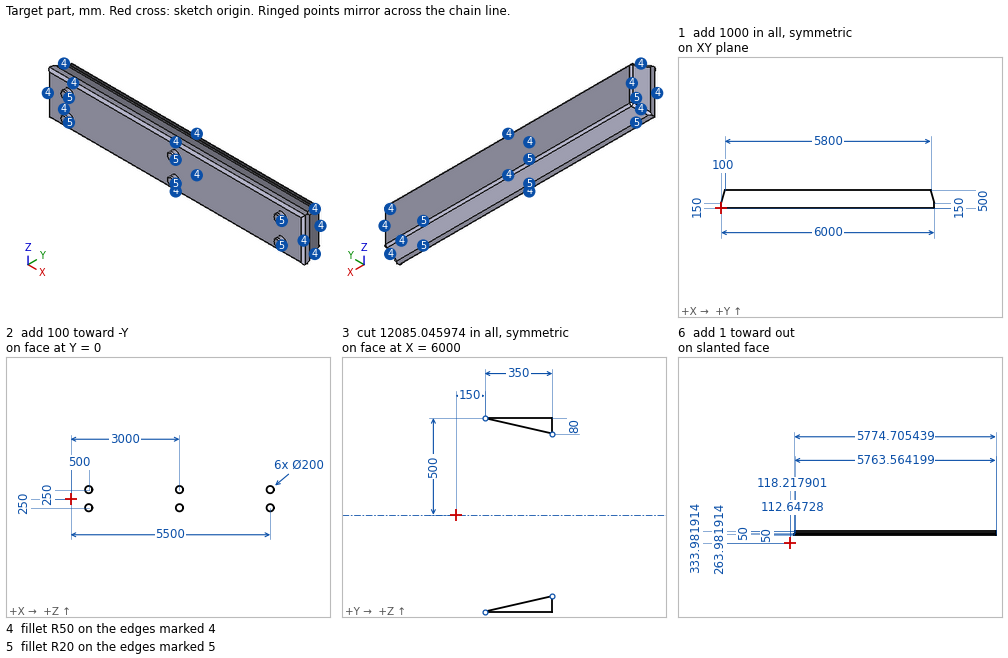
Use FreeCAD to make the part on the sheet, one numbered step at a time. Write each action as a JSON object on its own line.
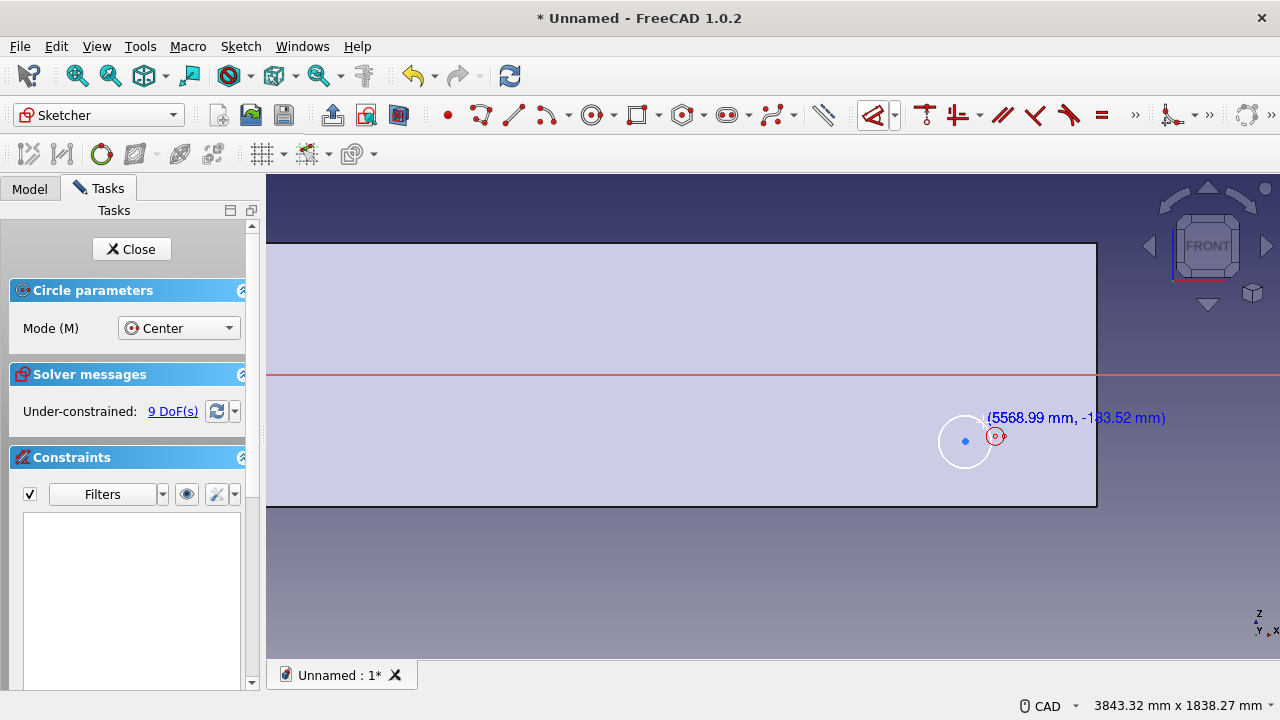
{"action": "left_click", "coordinate": [965, 309]}
{"action": "left_click", "coordinate": [983, 290]}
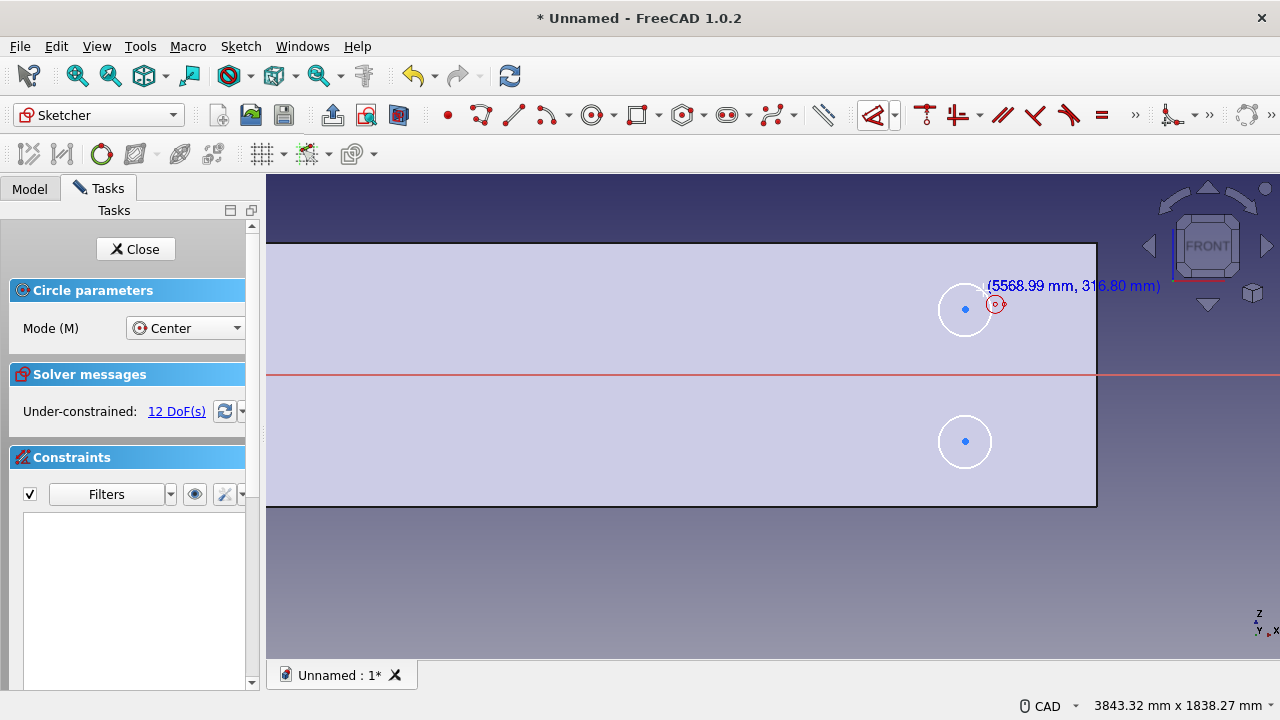
{"action": "left_click", "coordinate": [305, 309]}
{"action": "left_click", "coordinate": [324, 290]}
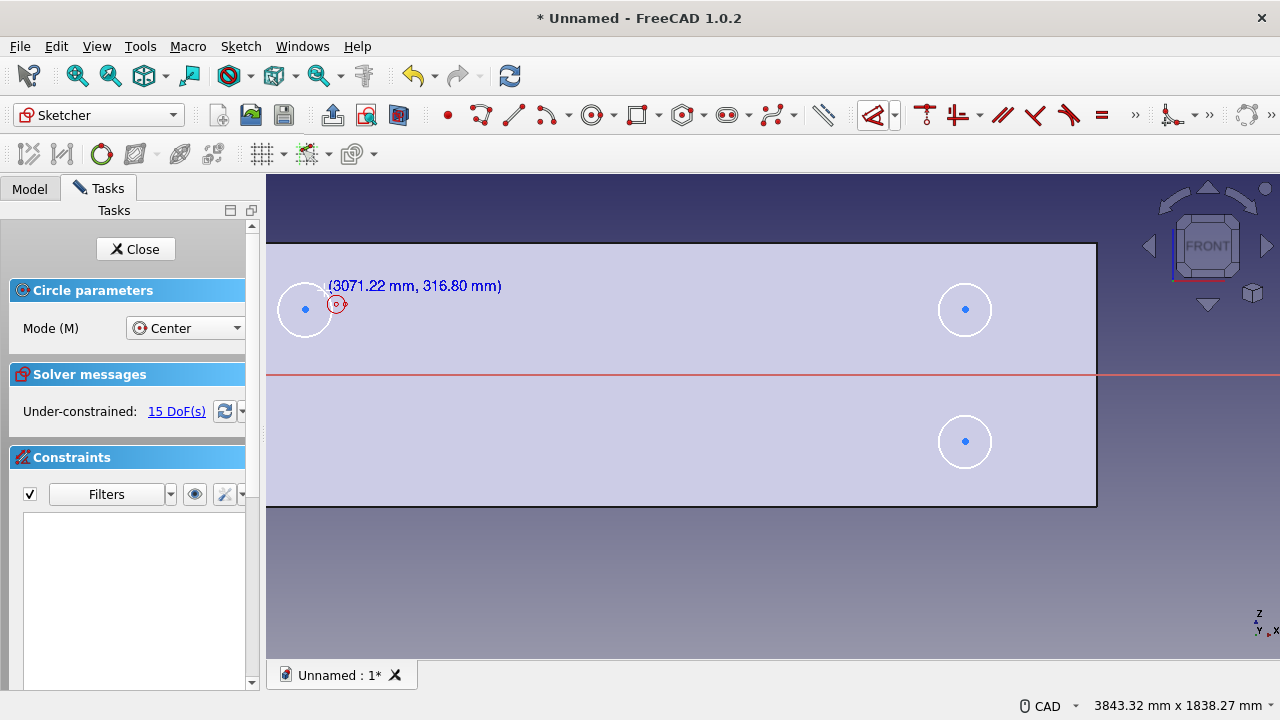
{"action": "left_click", "coordinate": [305, 441]}
{"action": "left_click", "coordinate": [324, 422]}
{"action": "key", "text": "Escape"}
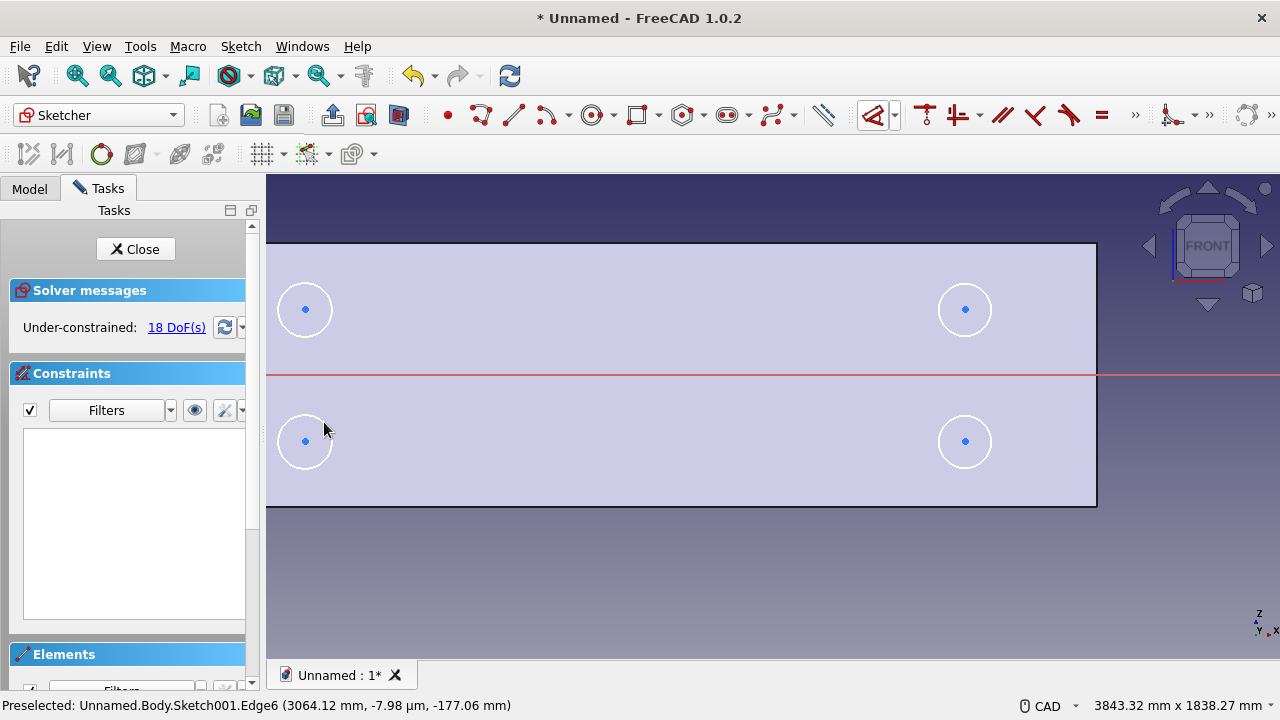
{"action": "scroll", "coordinate": [968, 441], "scroll_direction": "down", "scroll_amount": 5}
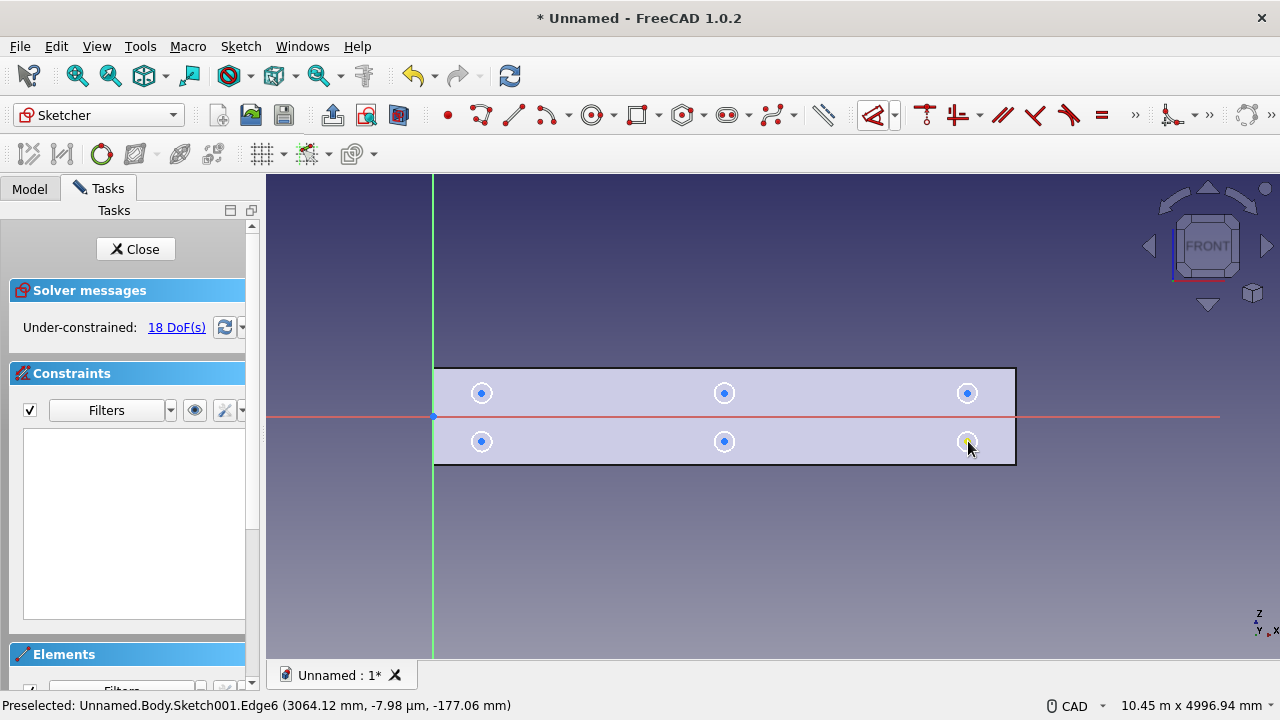
{"action": "scroll", "coordinate": [489, 386], "scroll_direction": "up", "scroll_amount": 2}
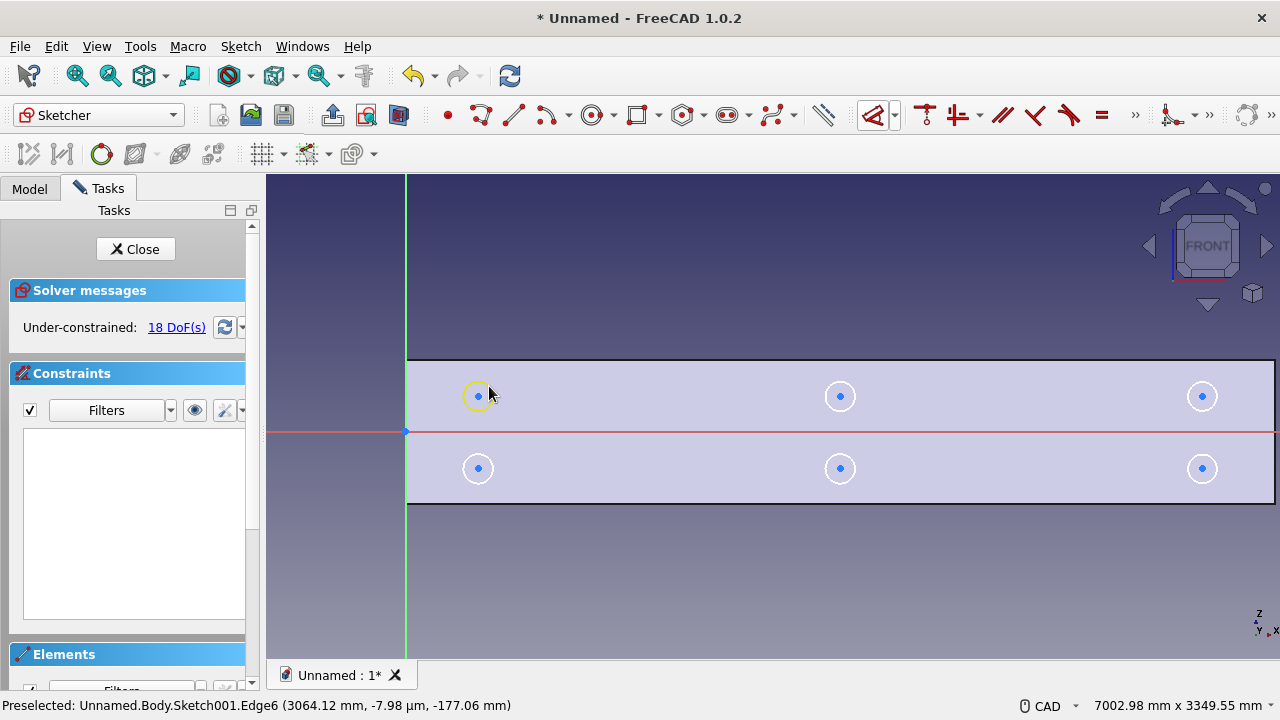
{"action": "left_click", "coordinate": [489, 386]}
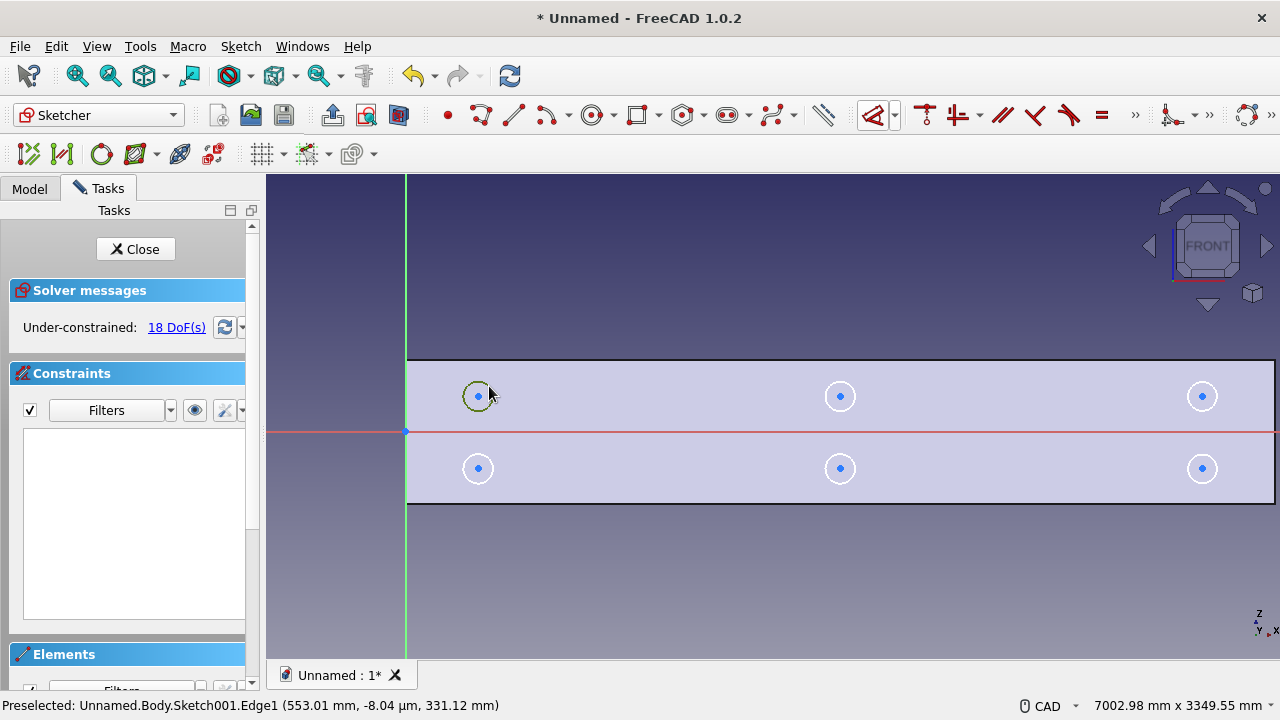
{"action": "left_click", "coordinate": [489, 458]}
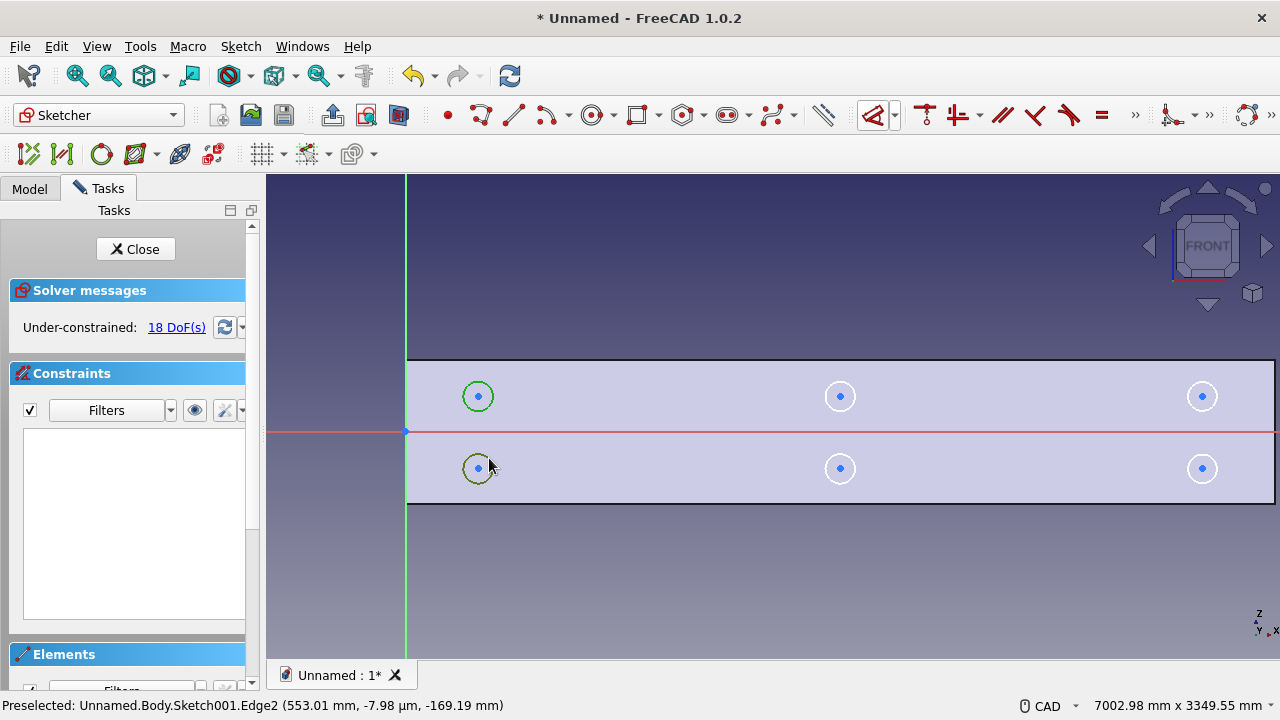
{"action": "scroll", "coordinate": [487, 385], "scroll_direction": "down", "scroll_amount": 2}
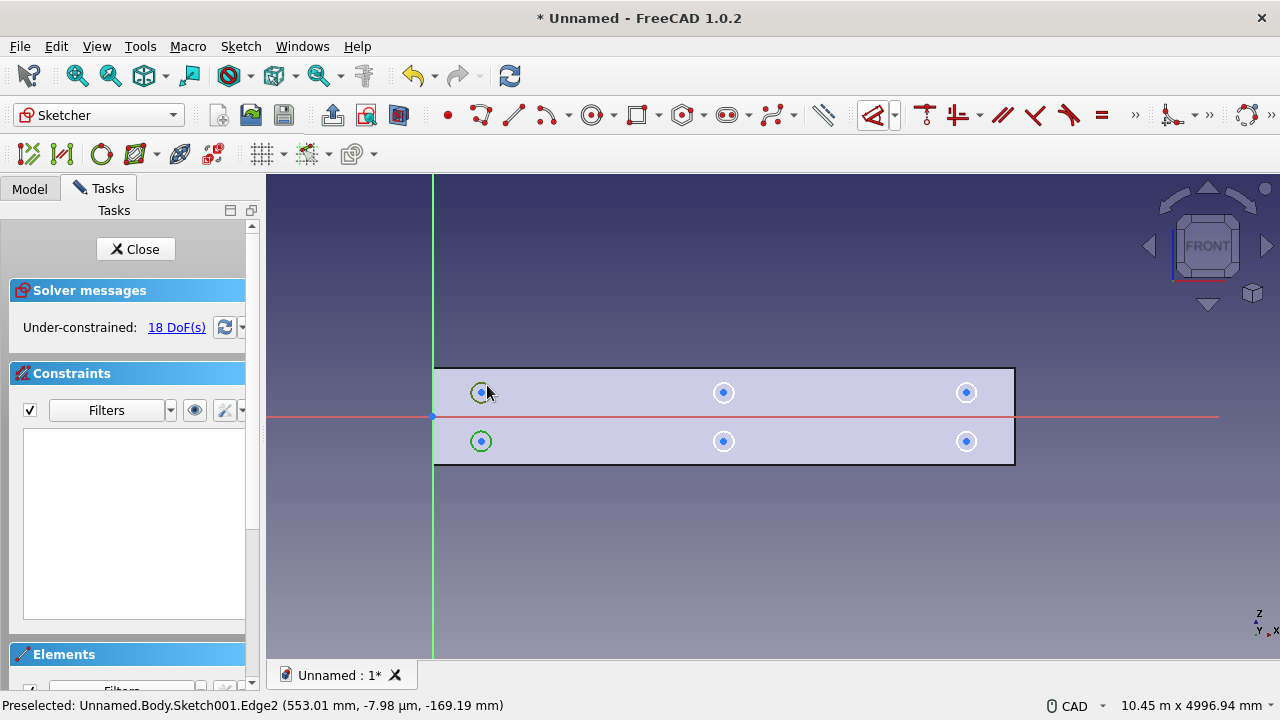
{"action": "scroll", "coordinate": [973, 435], "scroll_direction": "up", "scroll_amount": 2}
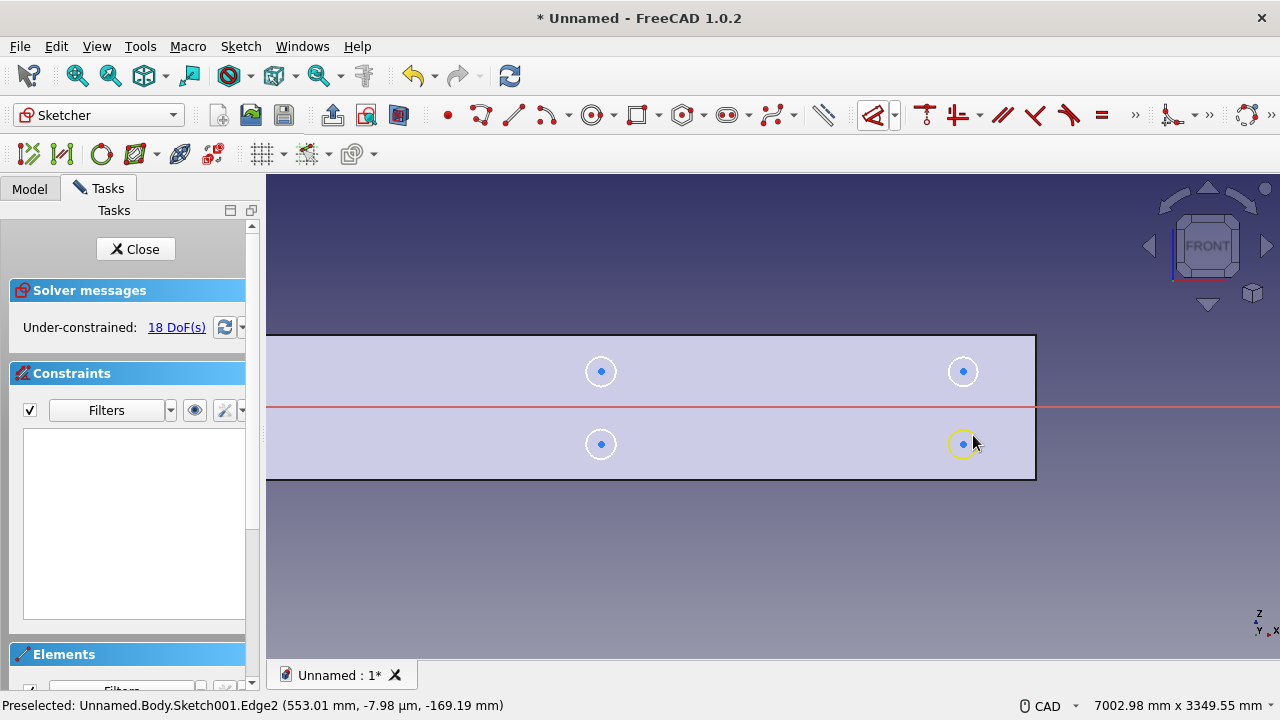
{"action": "left_click", "coordinate": [973, 434]}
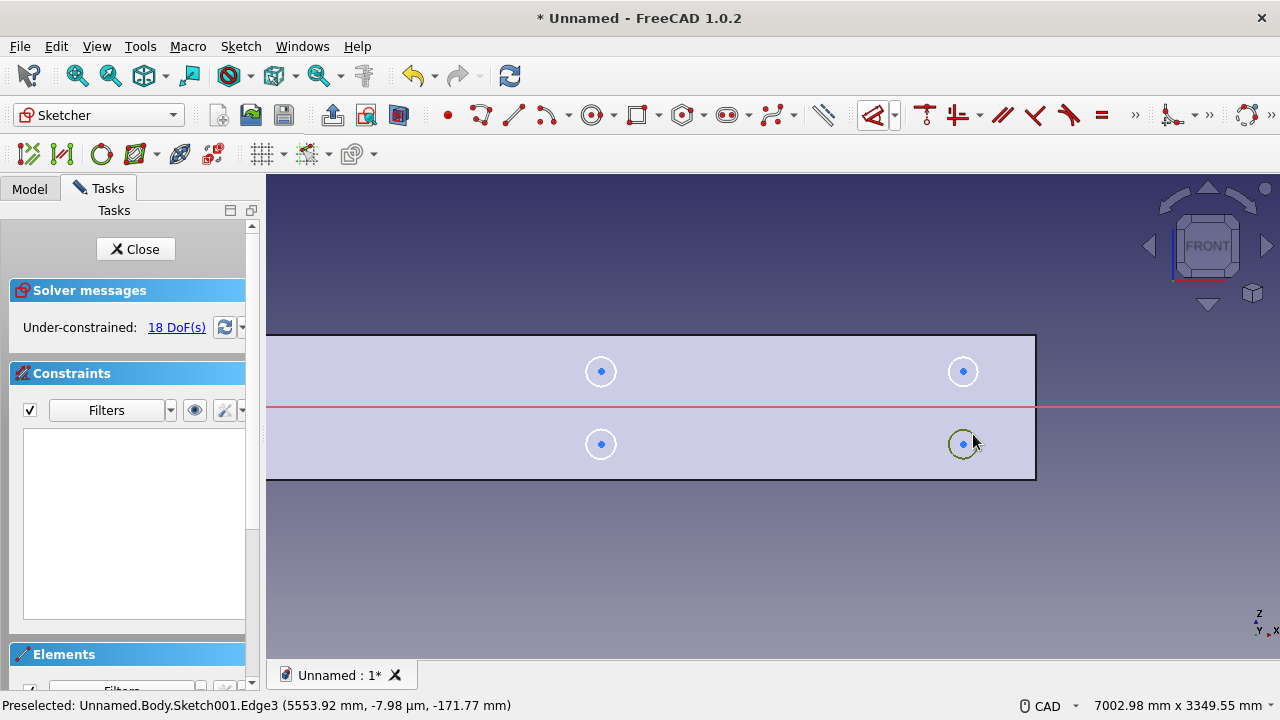
{"action": "left_click", "coordinate": [973, 362]}